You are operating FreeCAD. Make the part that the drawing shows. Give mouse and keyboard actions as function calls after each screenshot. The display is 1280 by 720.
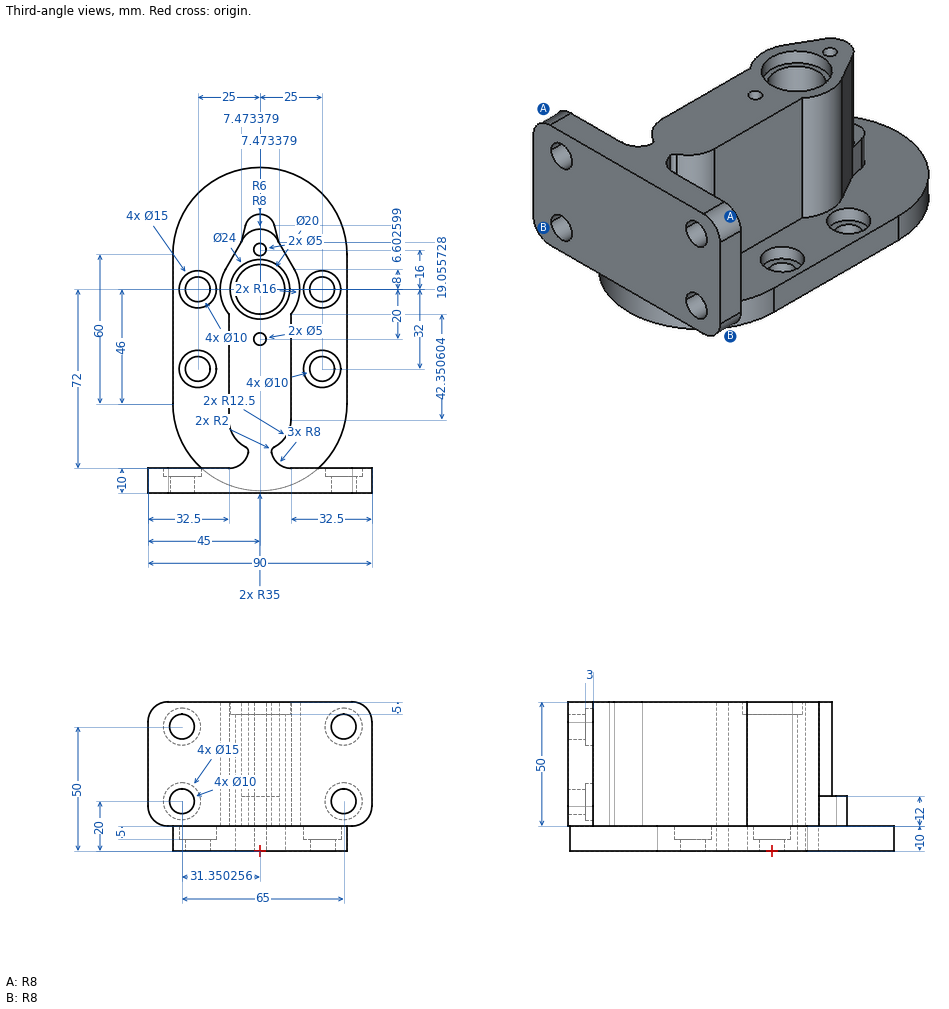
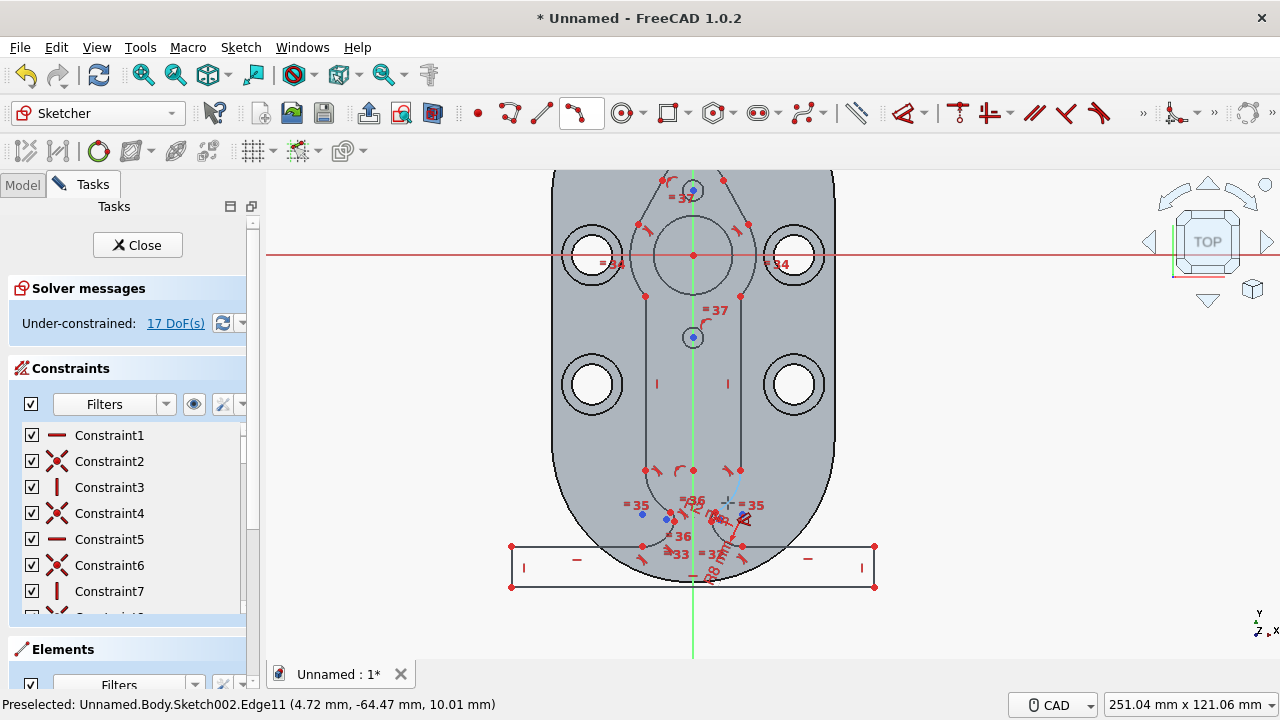
click(728, 503)
click(770, 490)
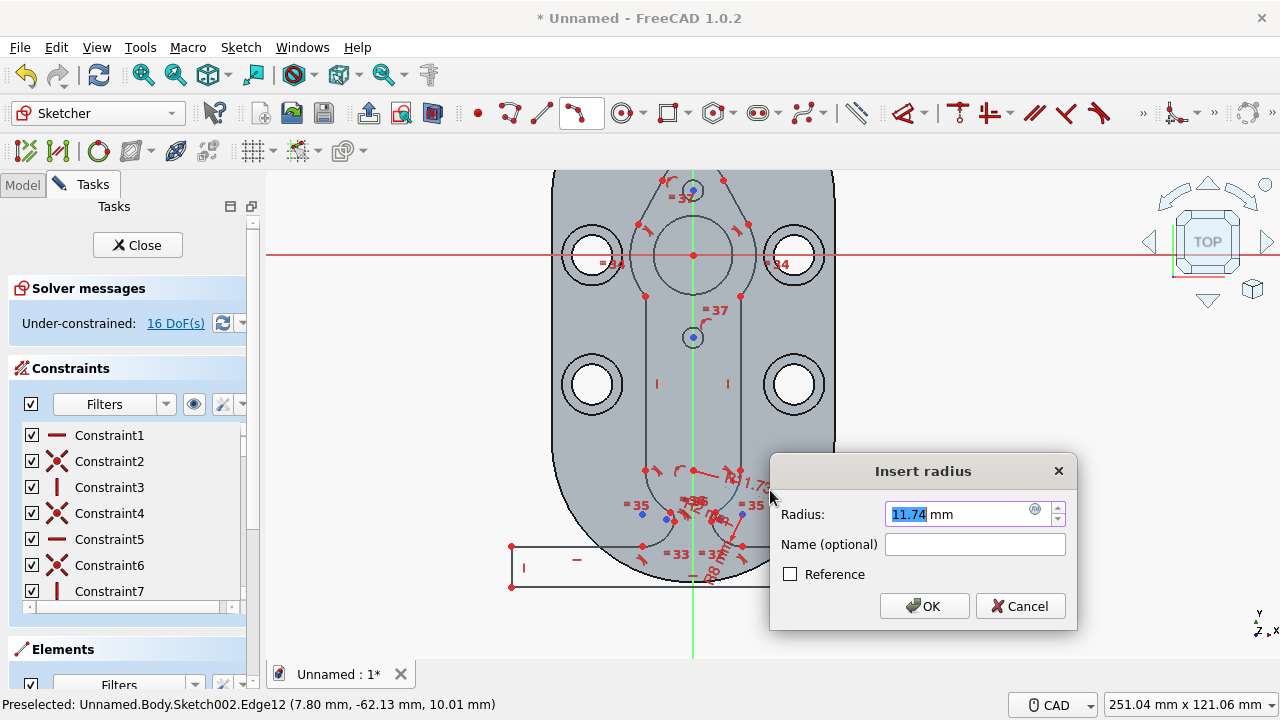
text(12.5)
key(Return)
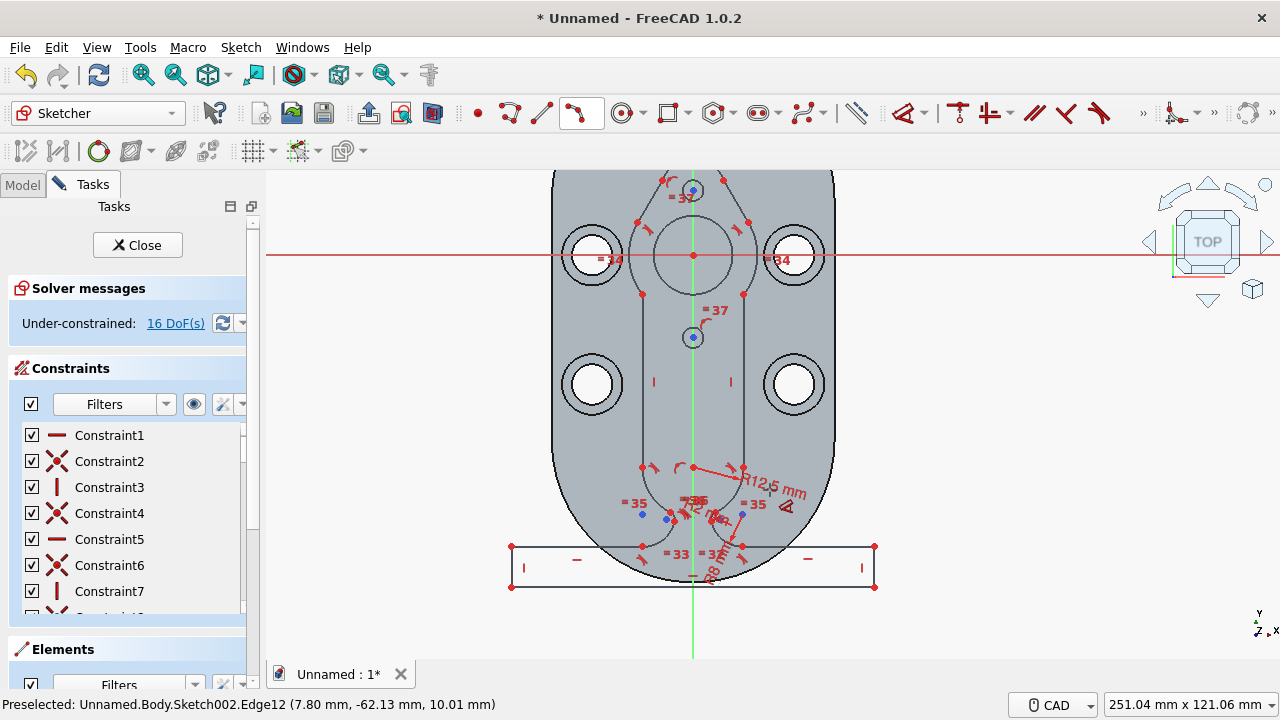
click(754, 275)
click(784, 285)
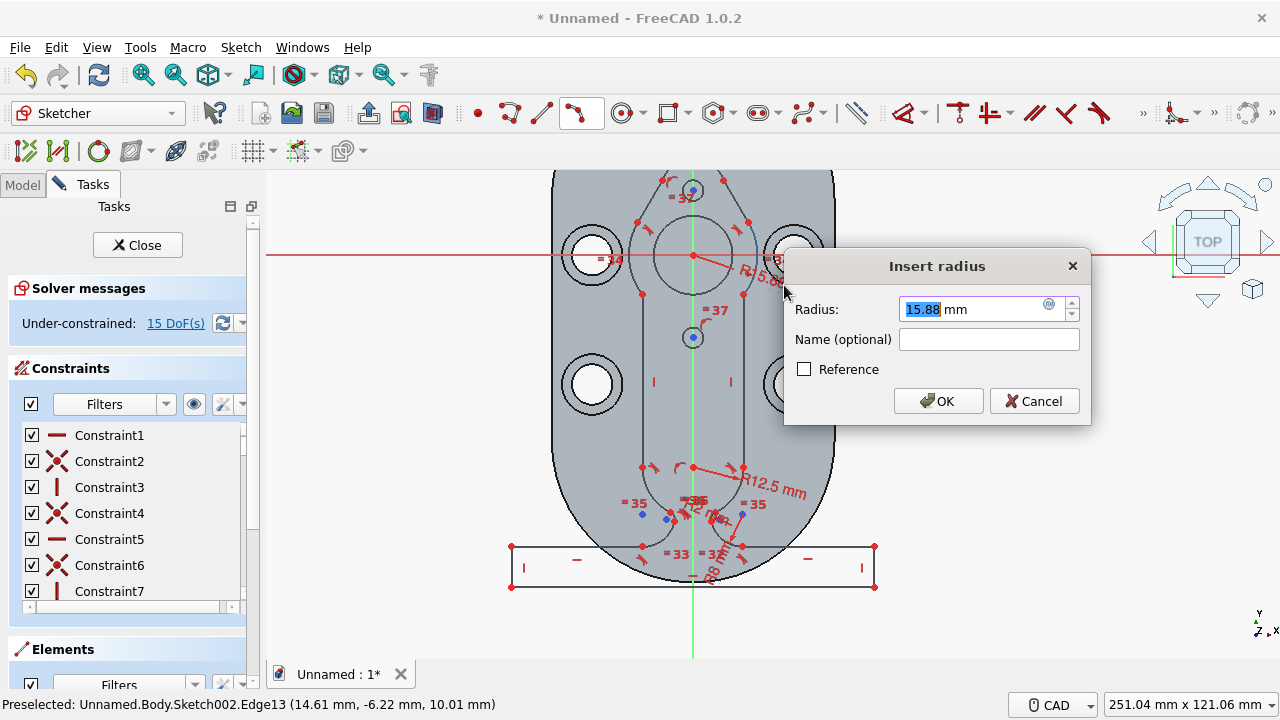
text(16)
key(Return)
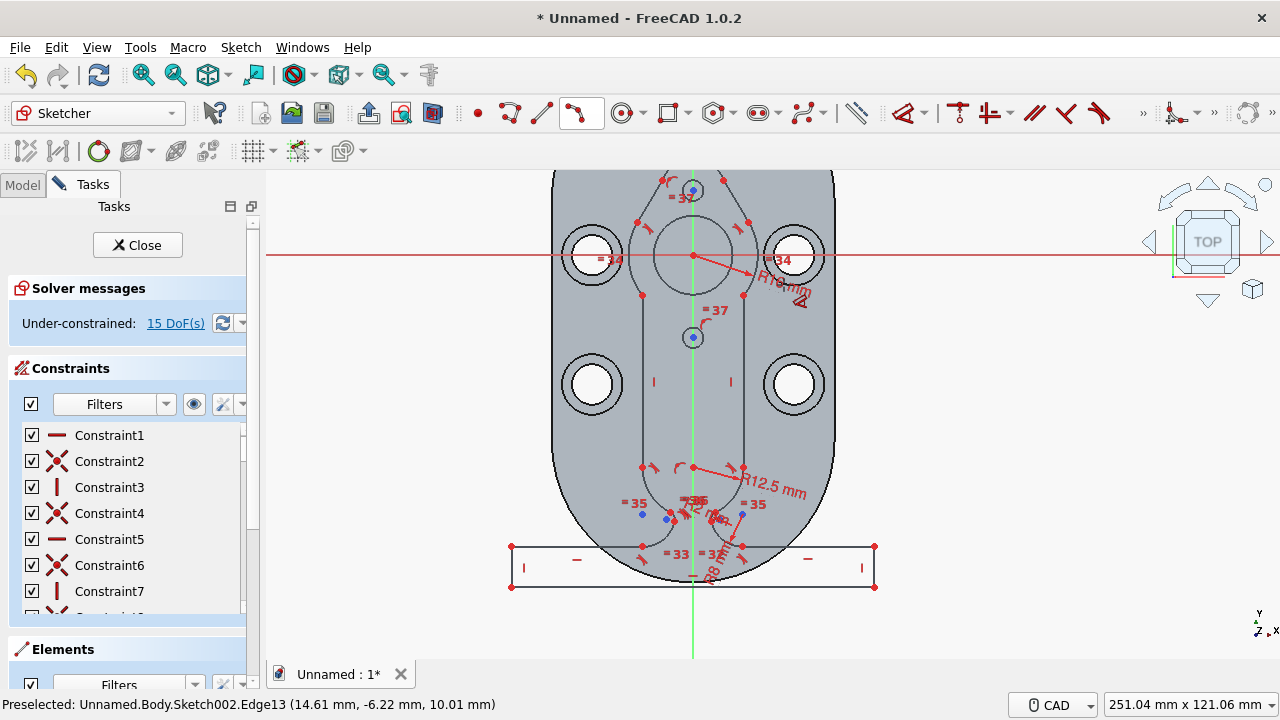
scroll(693, 328, up, 4)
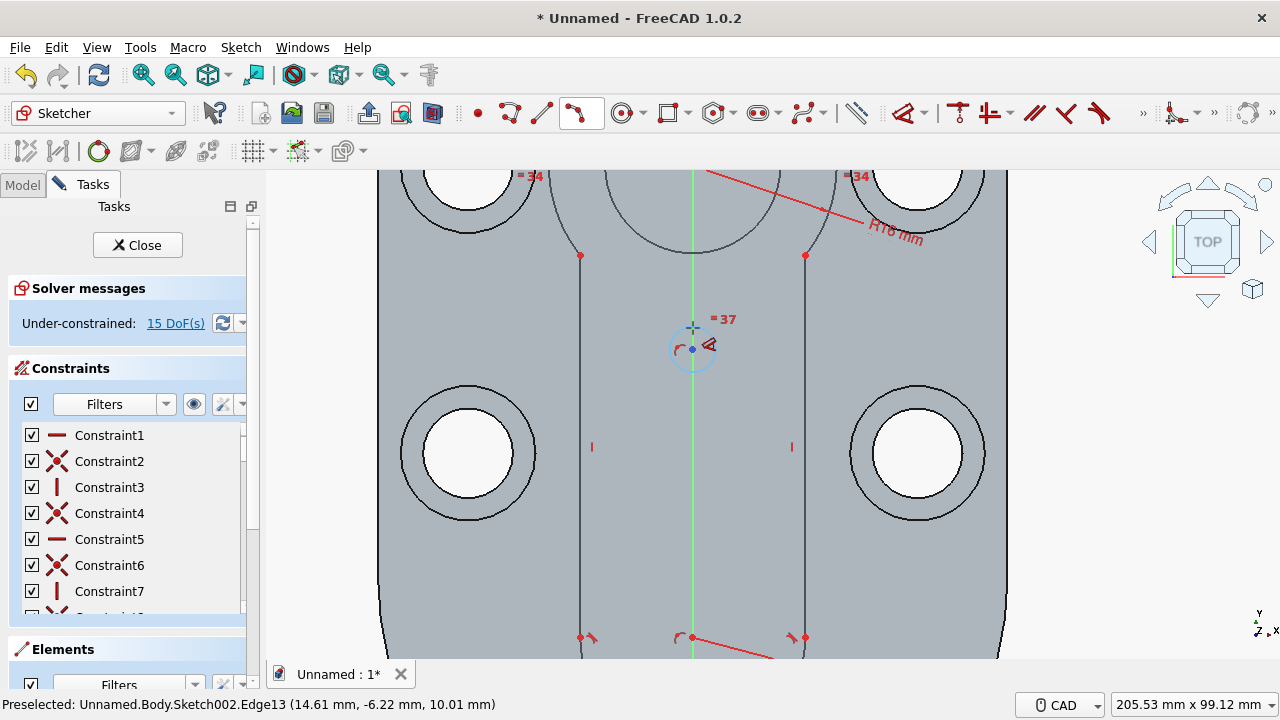
click(693, 327)
click(719, 302)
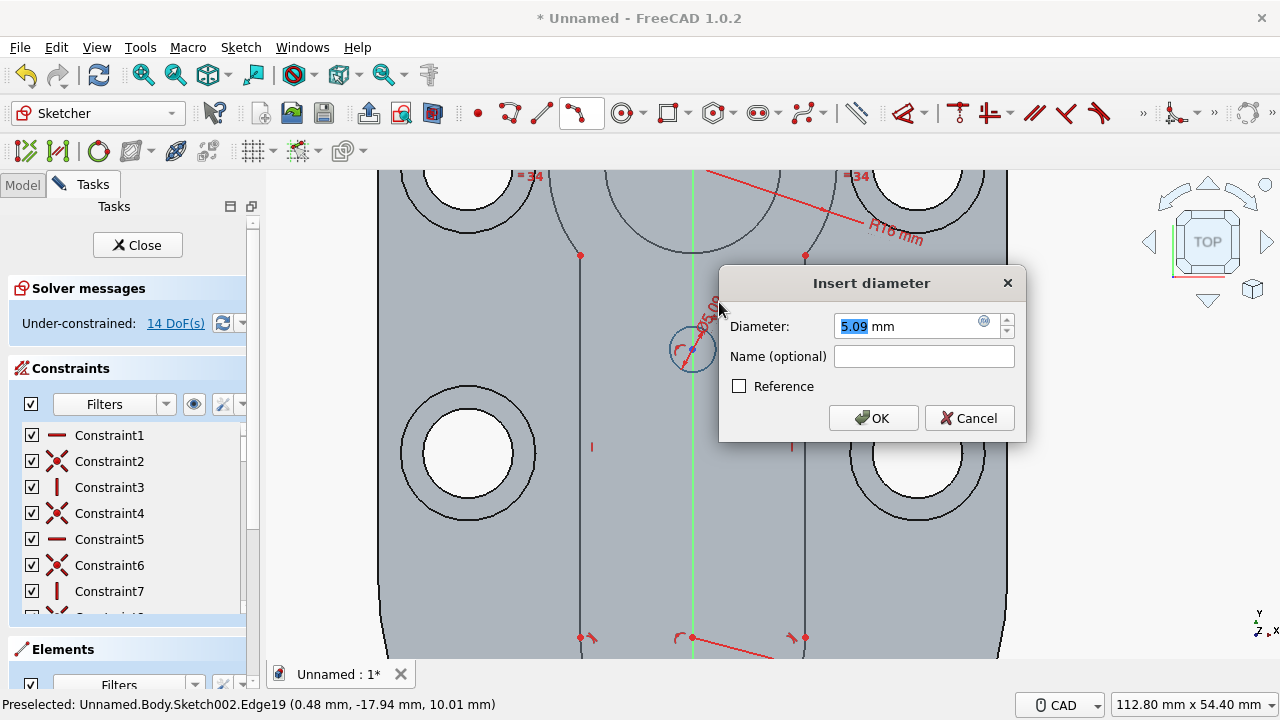
text(5)
key(Return)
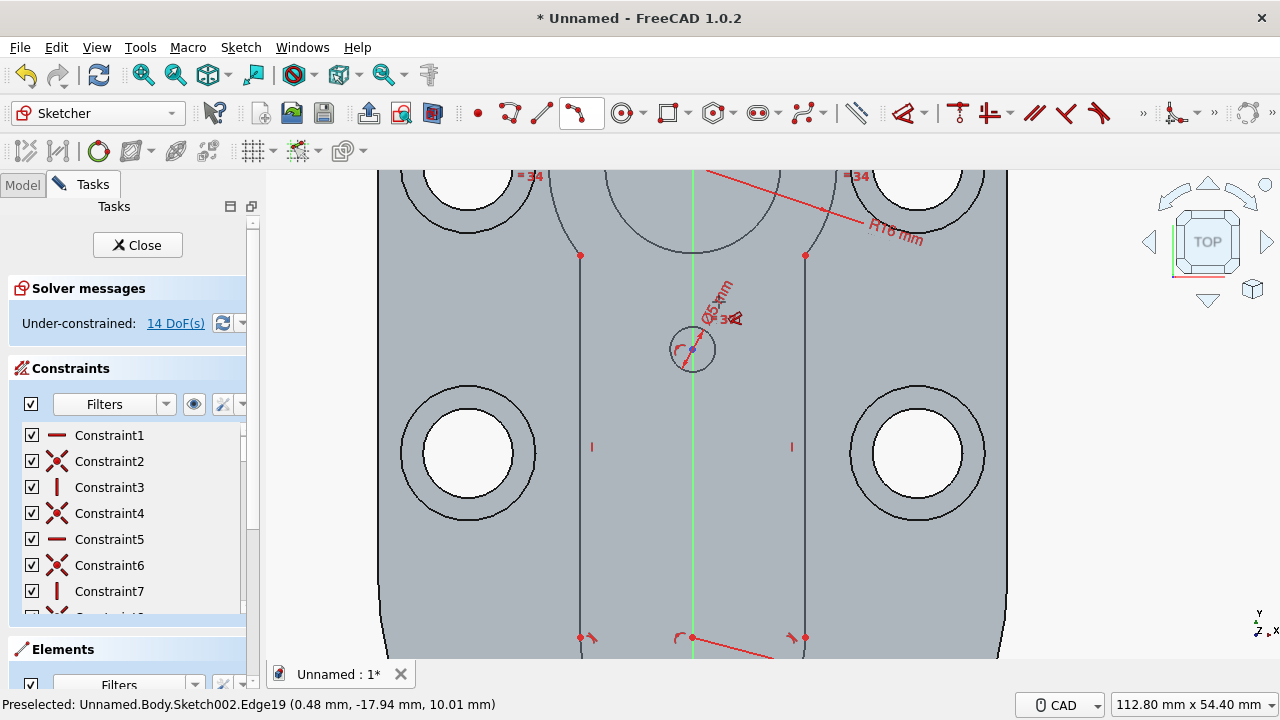
click(631, 228)
click(608, 251)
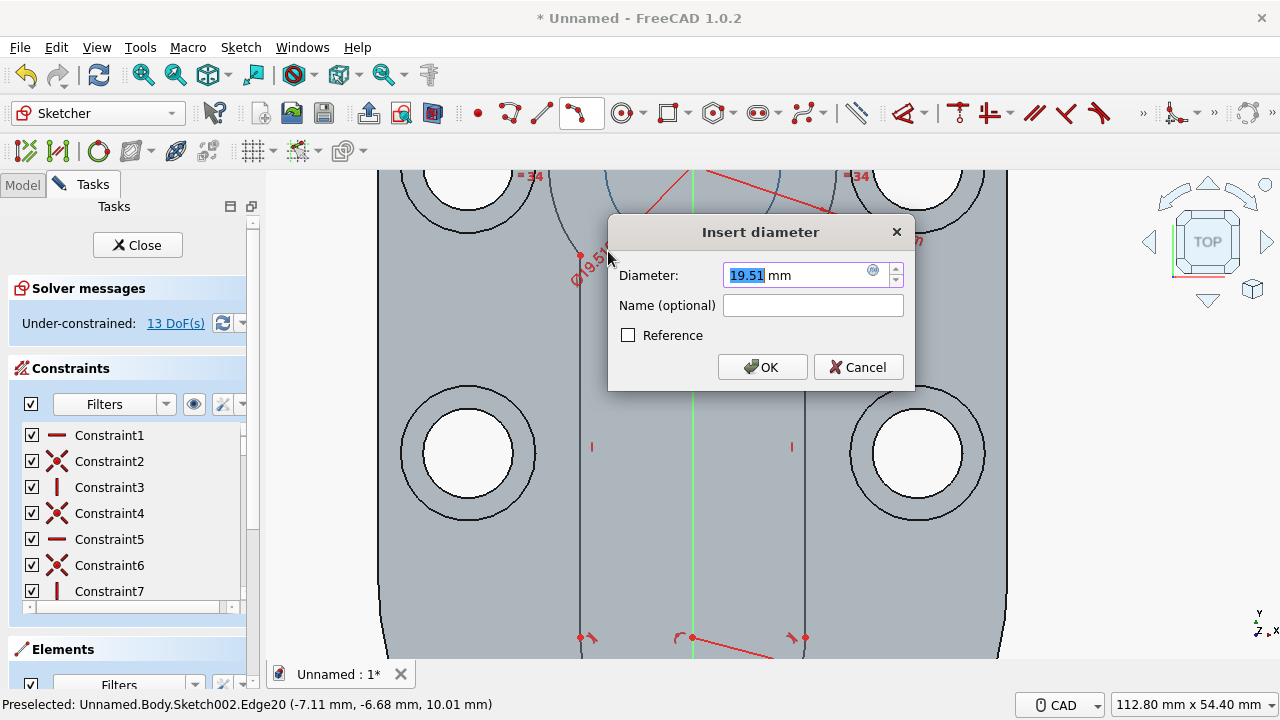
text(20)
key(Return)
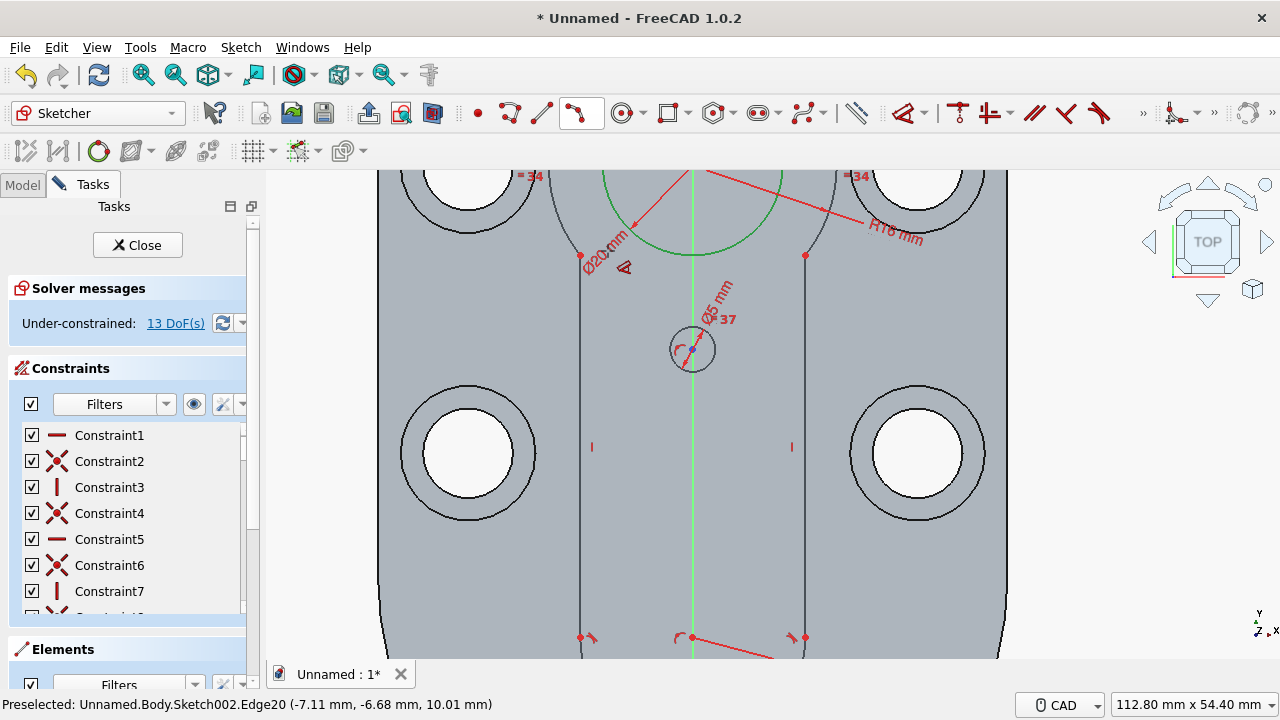
scroll(710, 410, down, 6)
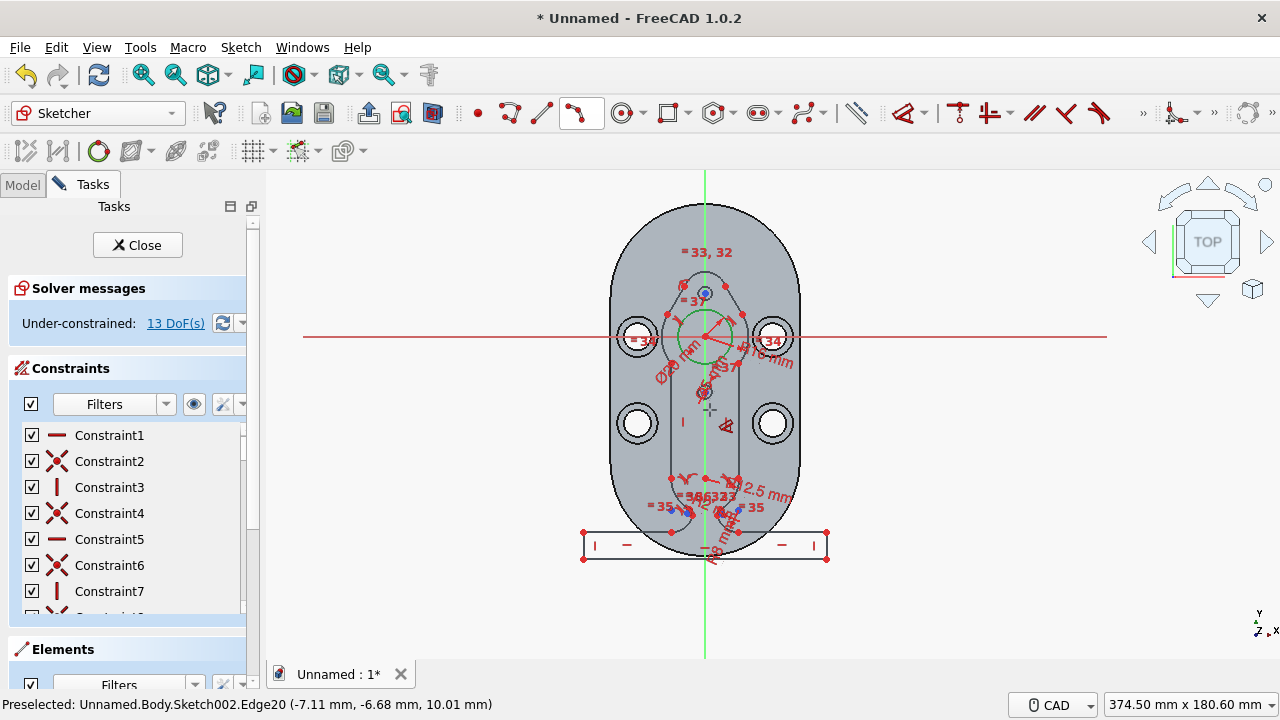
scroll(584, 540, up, 3)